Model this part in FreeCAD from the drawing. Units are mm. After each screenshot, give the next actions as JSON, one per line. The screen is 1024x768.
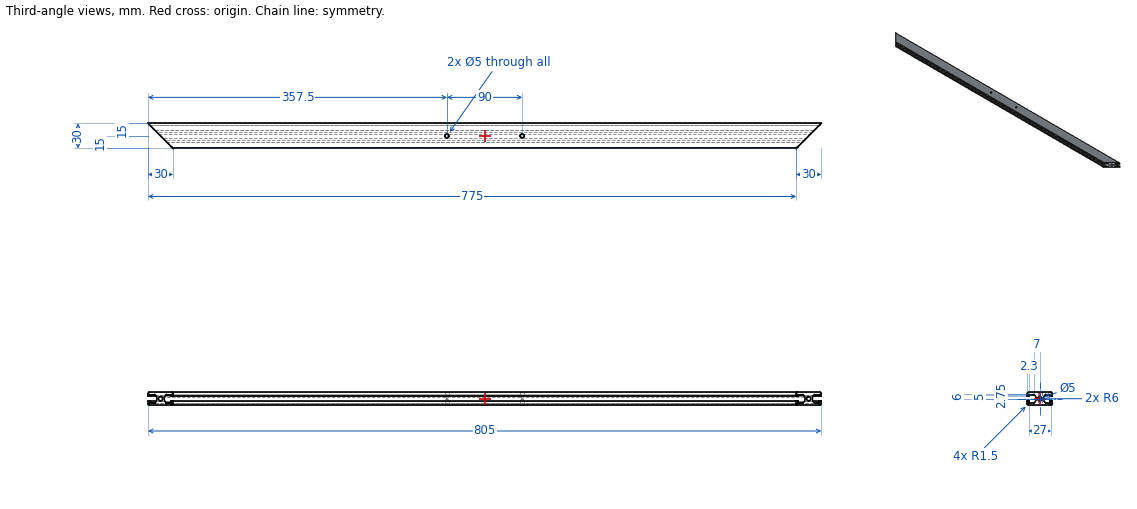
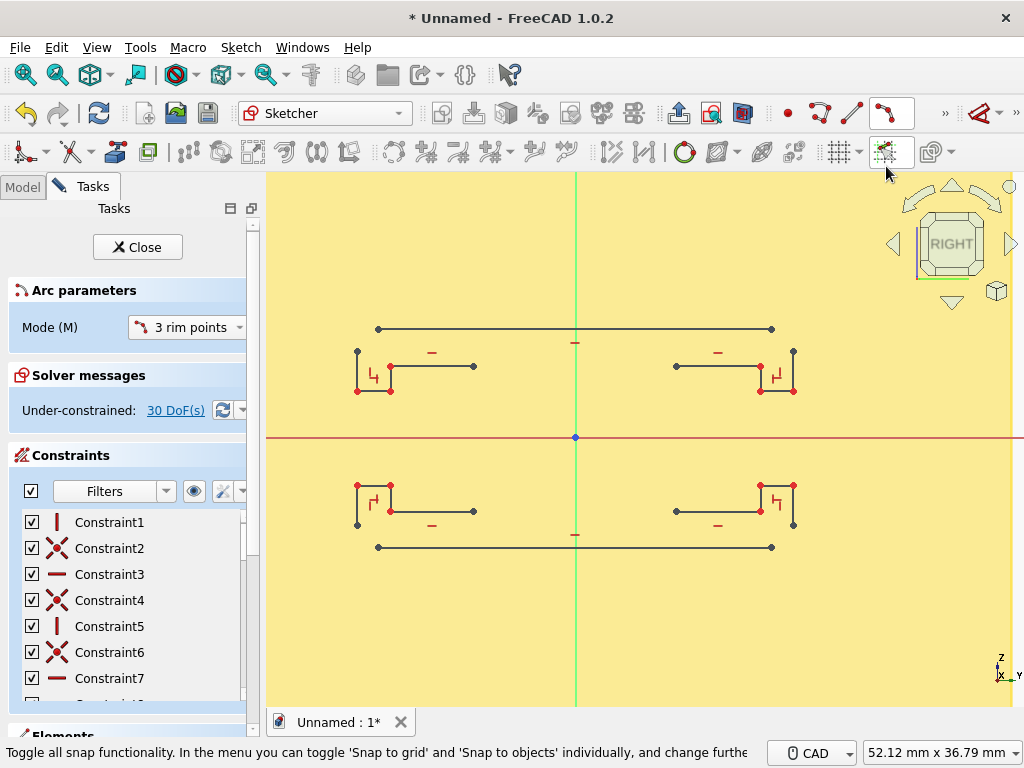
{"action": "left_click", "coordinate": [474, 366]}
{"action": "left_click", "coordinate": [474, 512]}
{"action": "left_click", "coordinate": [511, 455]}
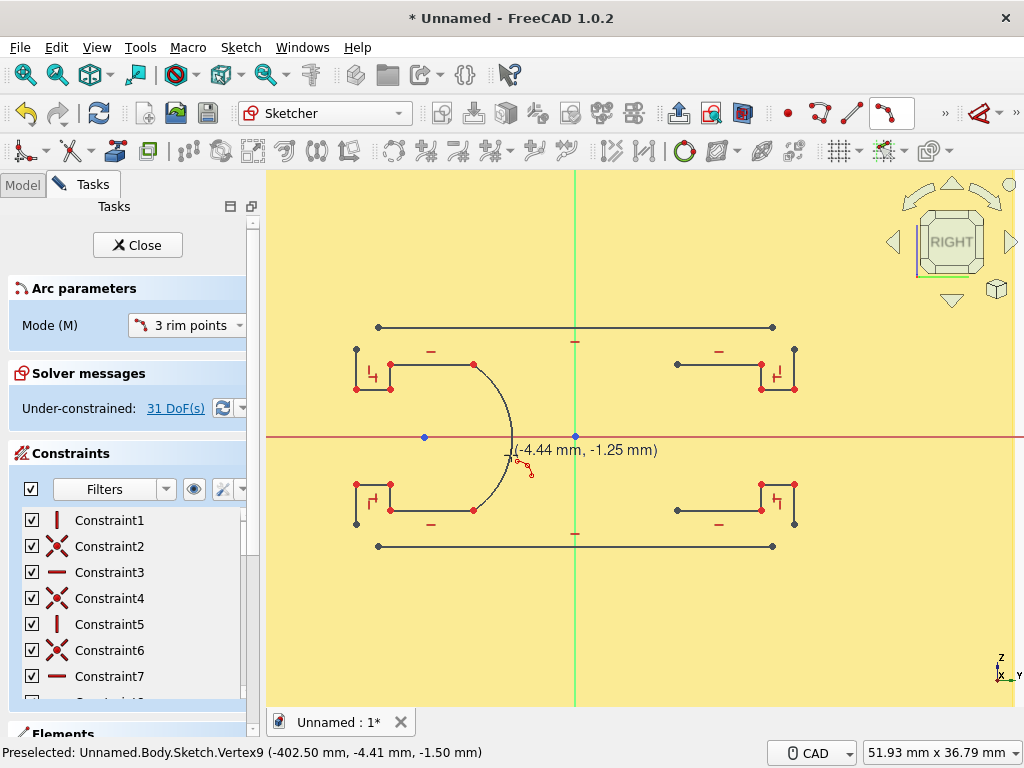
{"action": "left_click", "coordinate": [356, 525]}
{"action": "left_click", "coordinate": [378, 547]}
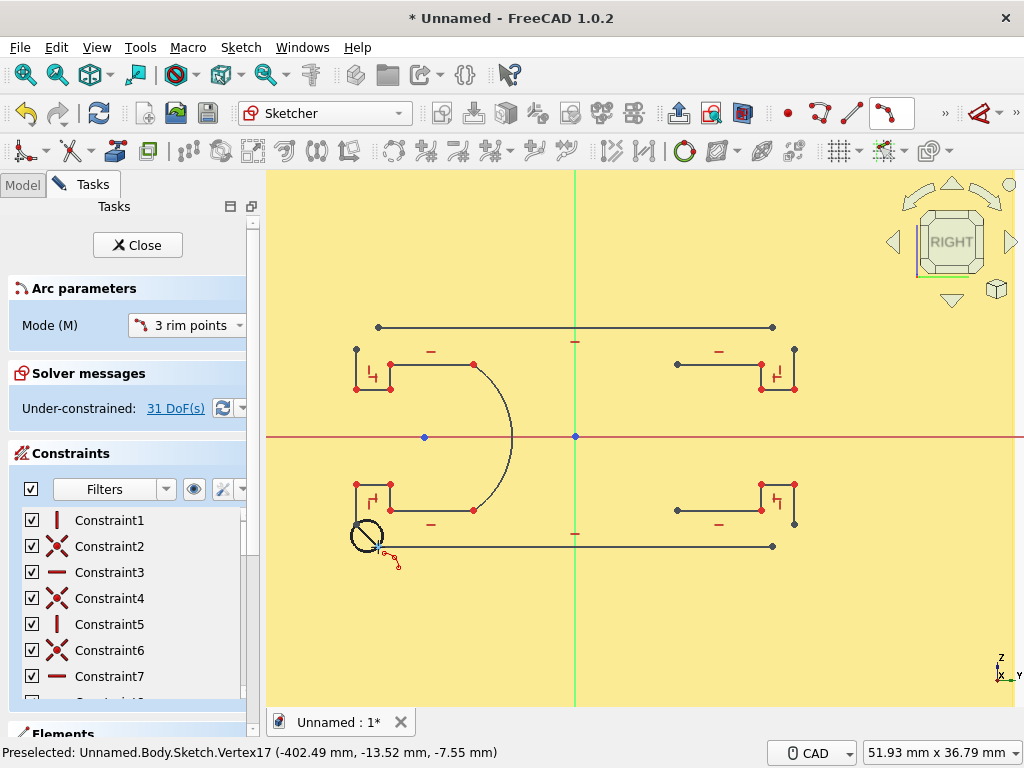
{"action": "scroll", "coordinate": [363, 540], "scroll_direction": "up", "scroll_amount": 5}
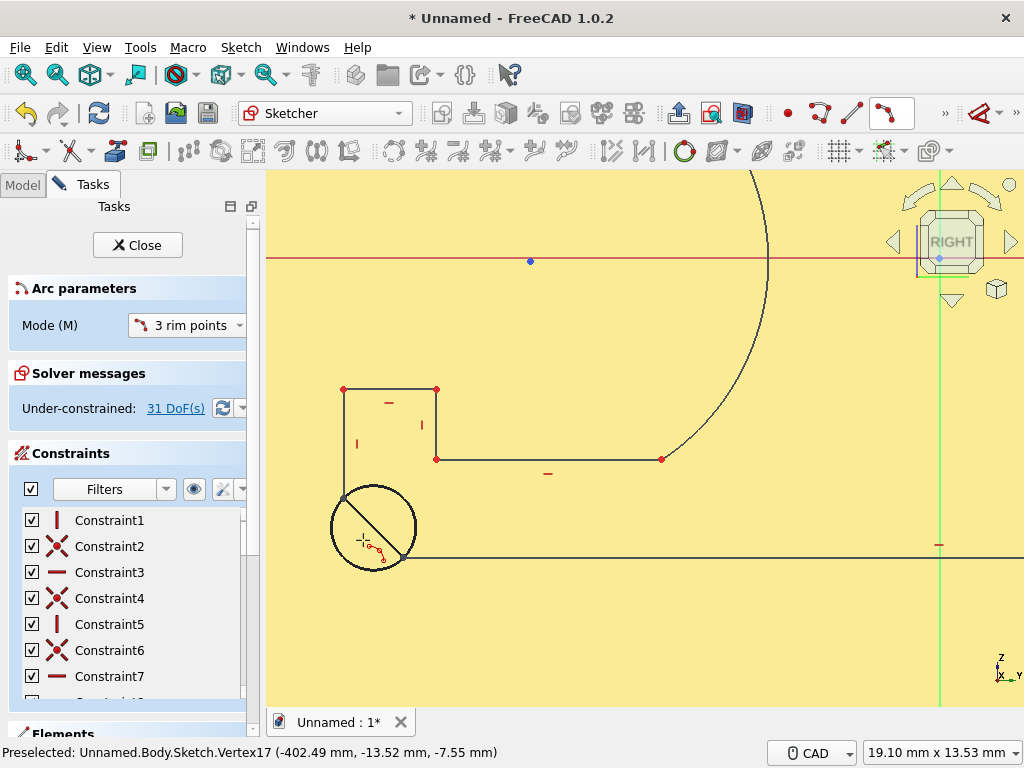
{"action": "left_click", "coordinate": [362, 538]}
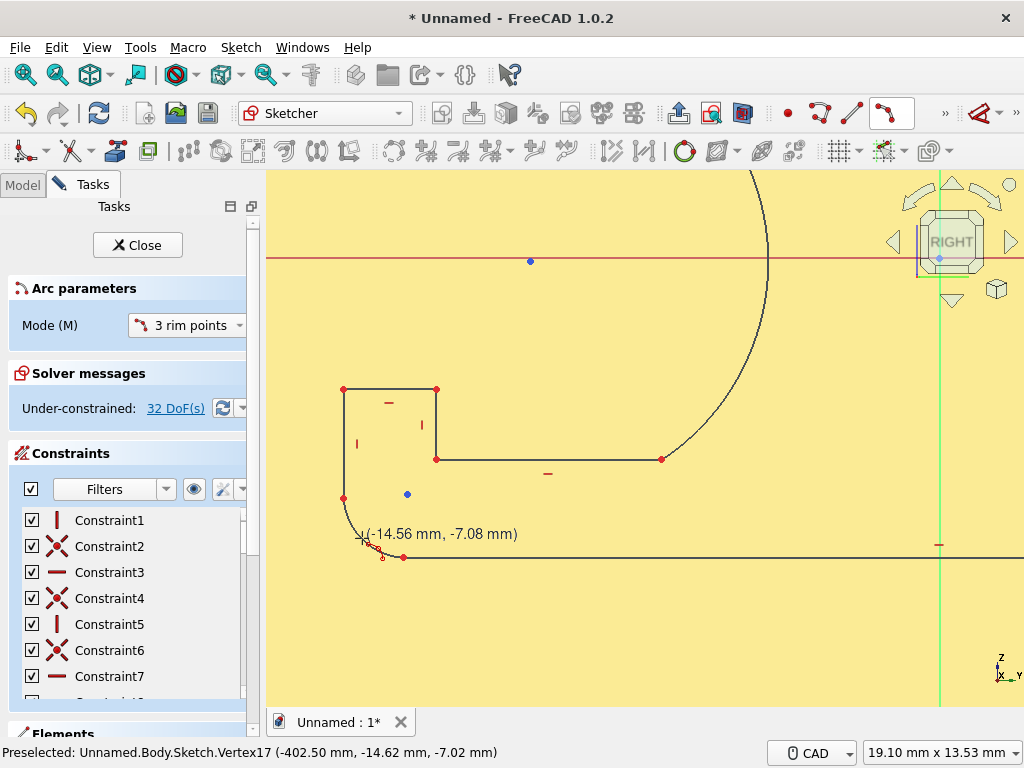
{"action": "scroll", "coordinate": [365, 543], "scroll_direction": "down", "scroll_amount": 5}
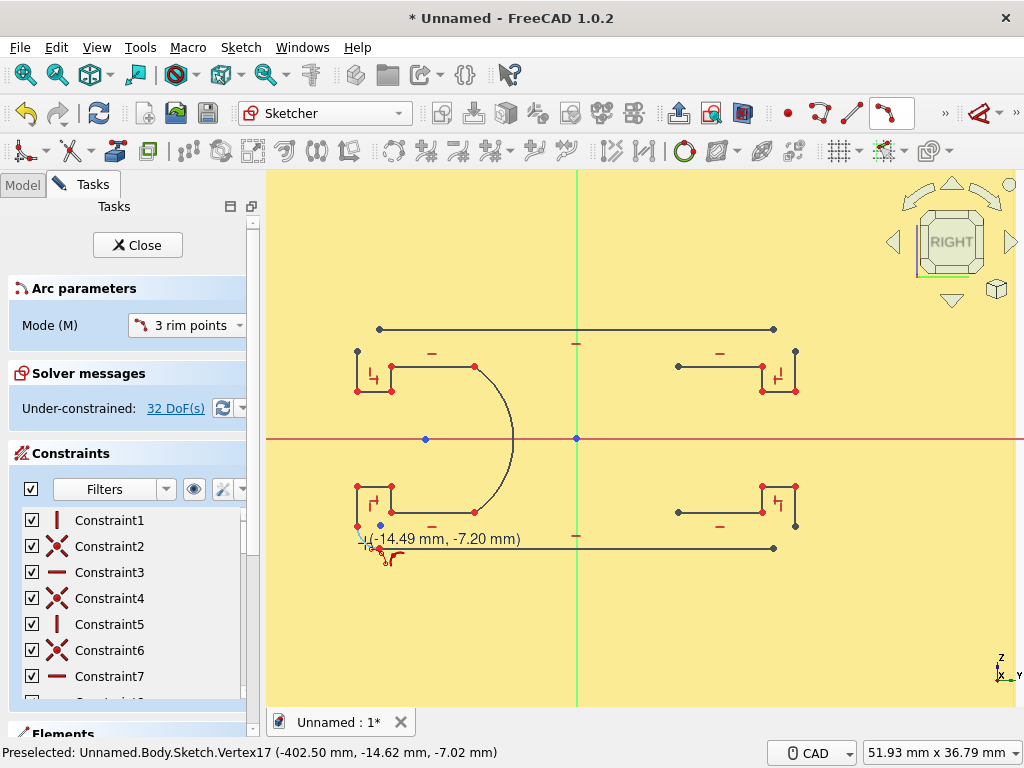
{"action": "left_click", "coordinate": [773, 549]}
{"action": "left_click", "coordinate": [795, 527]}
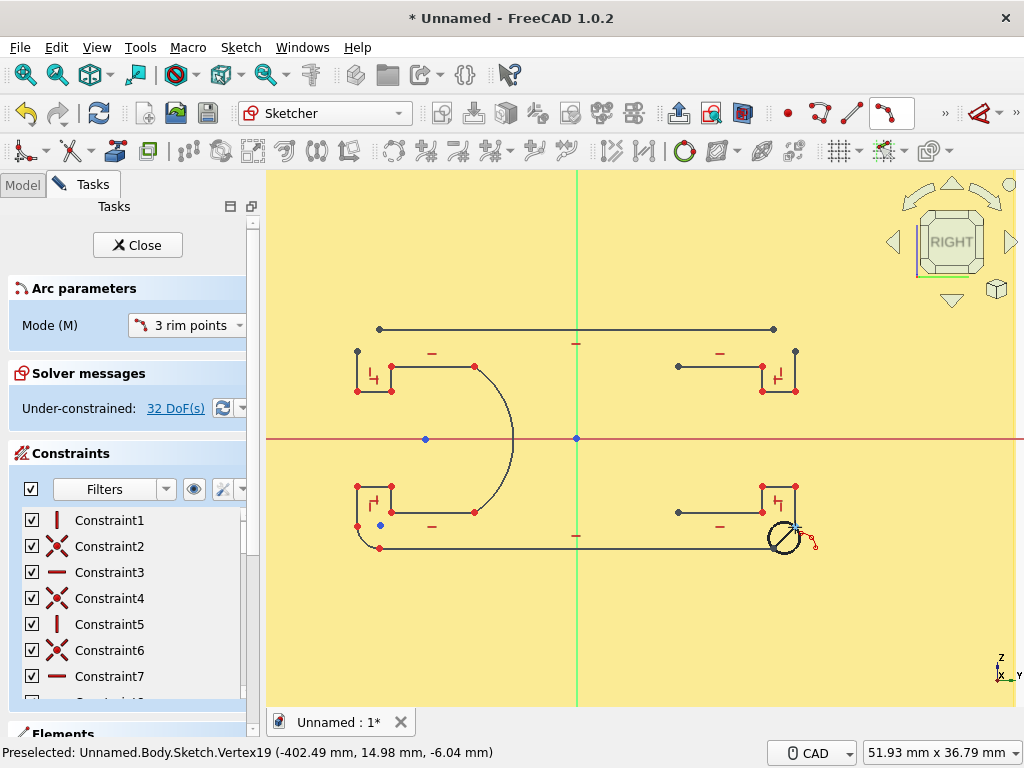
{"action": "scroll", "coordinate": [789, 542], "scroll_direction": "up", "scroll_amount": 5}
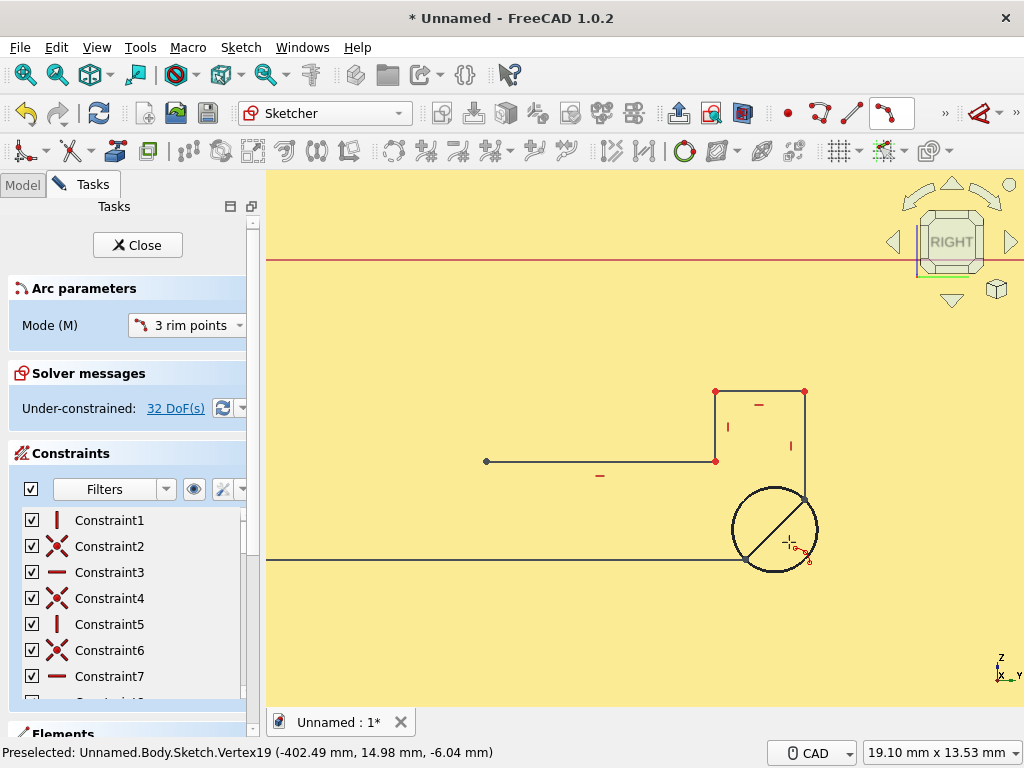
{"action": "left_click", "coordinate": [788, 540]}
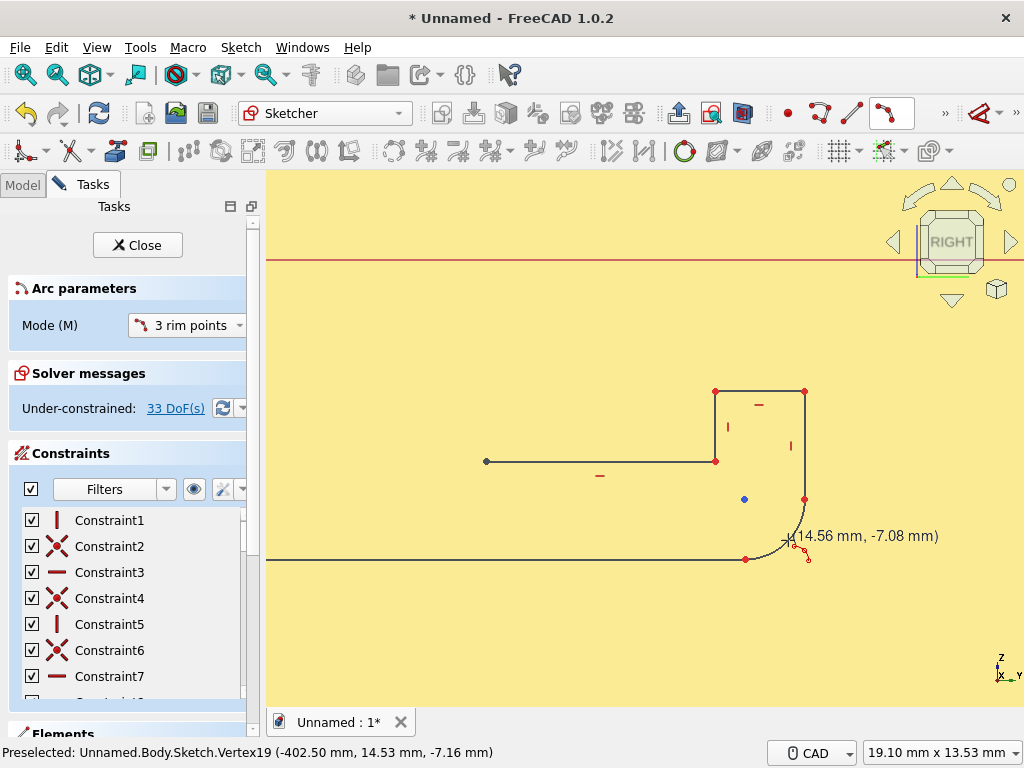
{"action": "left_click", "coordinate": [487, 462]}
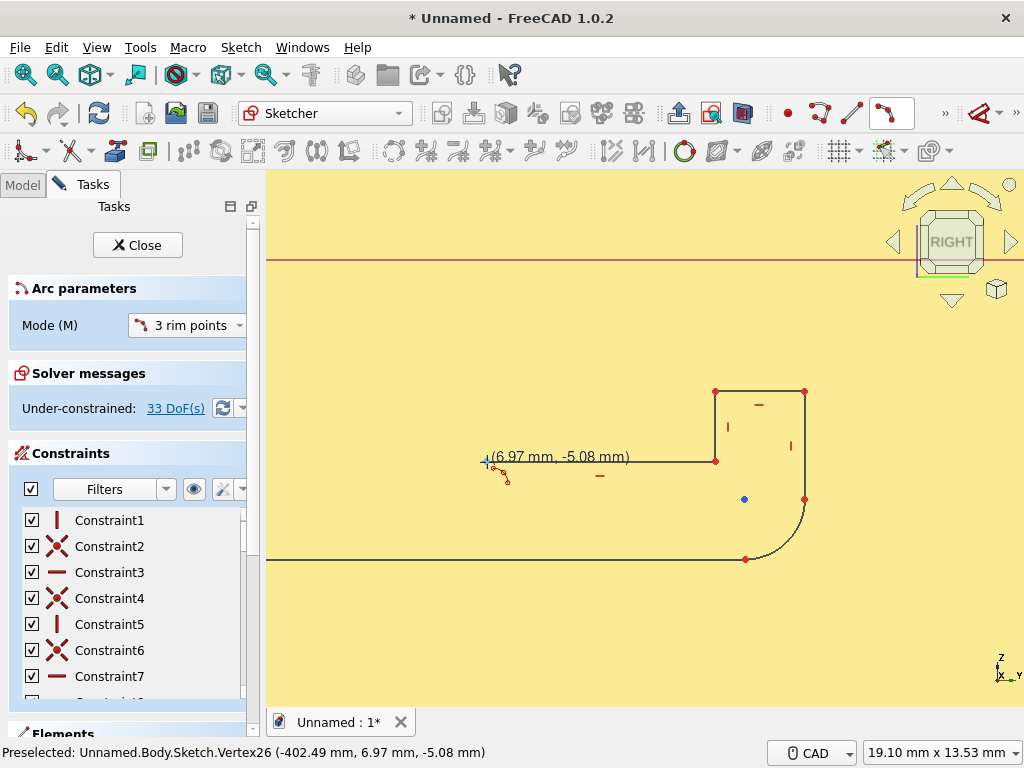
{"action": "scroll", "coordinate": [790, 542], "scroll_direction": "down", "scroll_amount": 5}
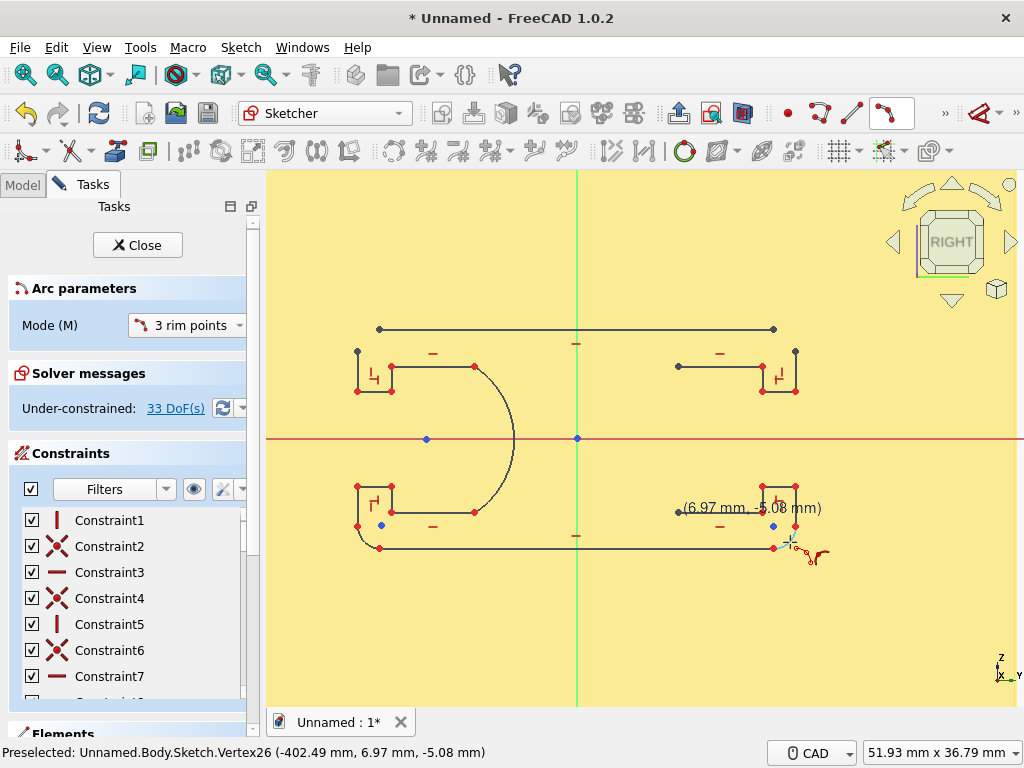
{"action": "left_click", "coordinate": [679, 367]}
{"action": "left_click", "coordinate": [642, 422]}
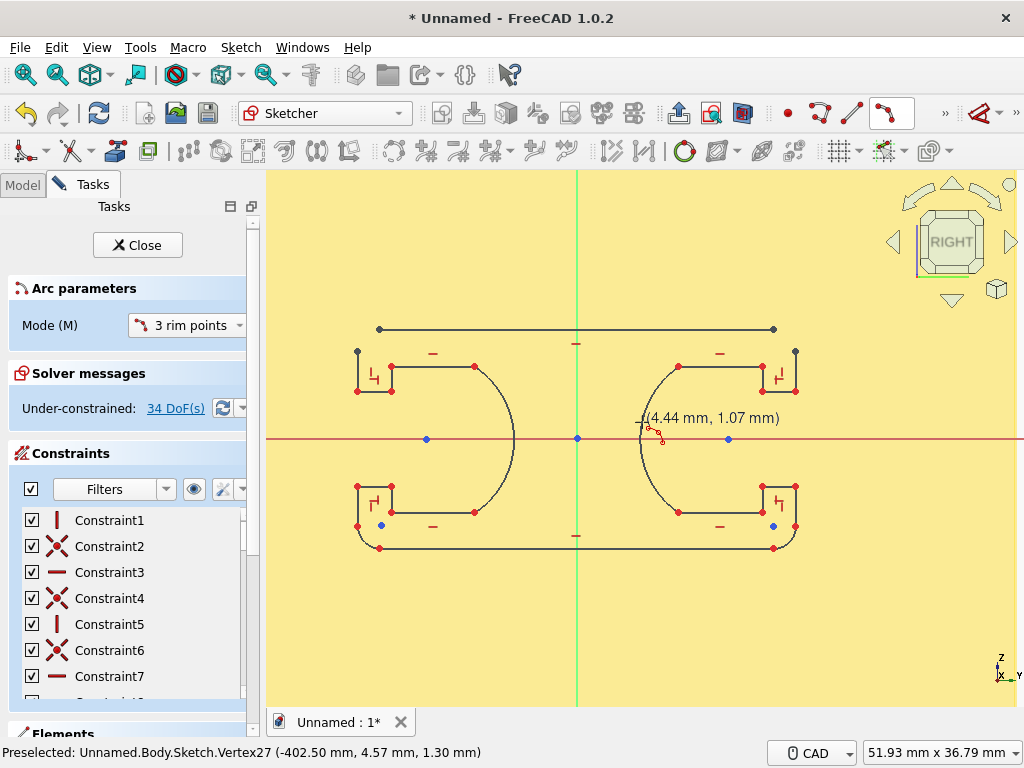
{"action": "left_click", "coordinate": [796, 352]}
{"action": "left_click", "coordinate": [774, 330]}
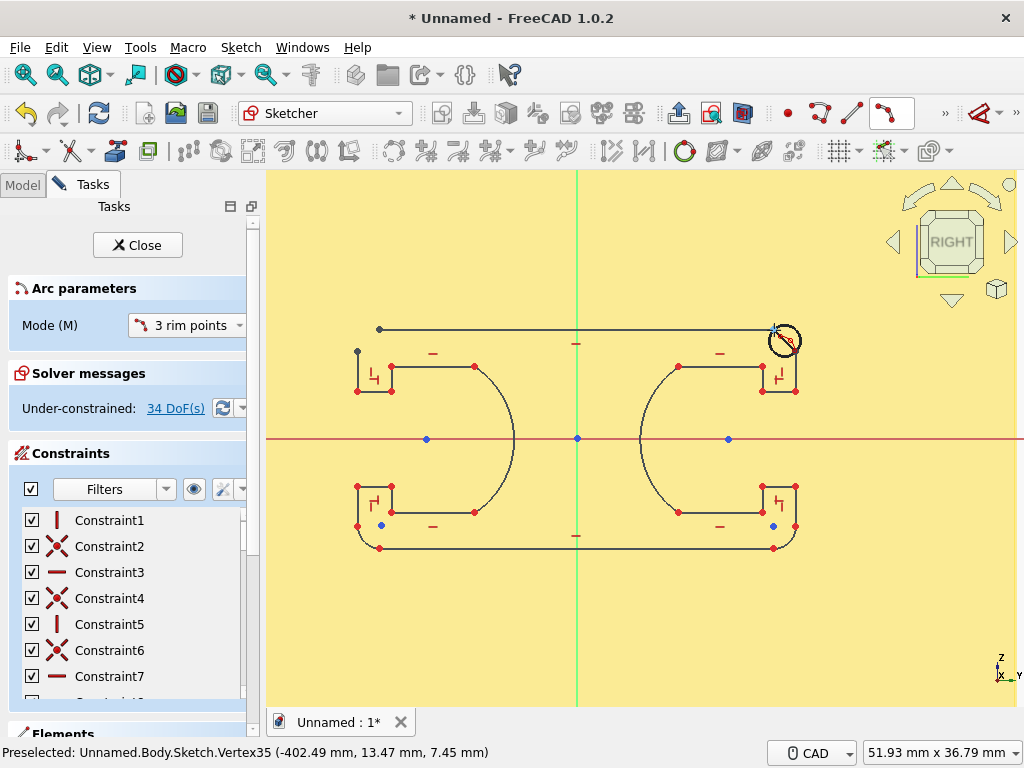
{"action": "scroll", "coordinate": [790, 336], "scroll_direction": "up", "scroll_amount": 5}